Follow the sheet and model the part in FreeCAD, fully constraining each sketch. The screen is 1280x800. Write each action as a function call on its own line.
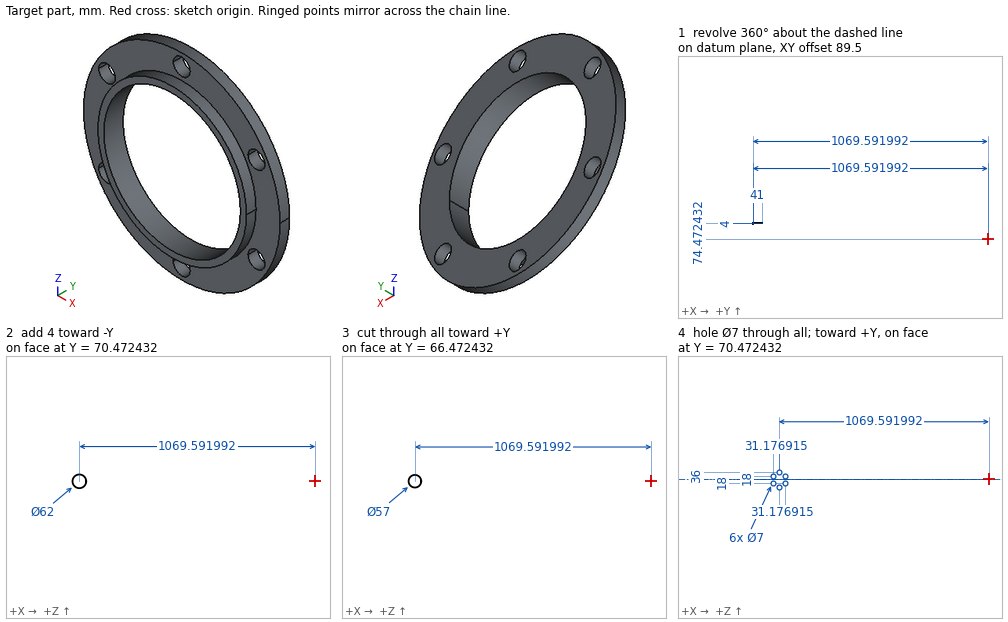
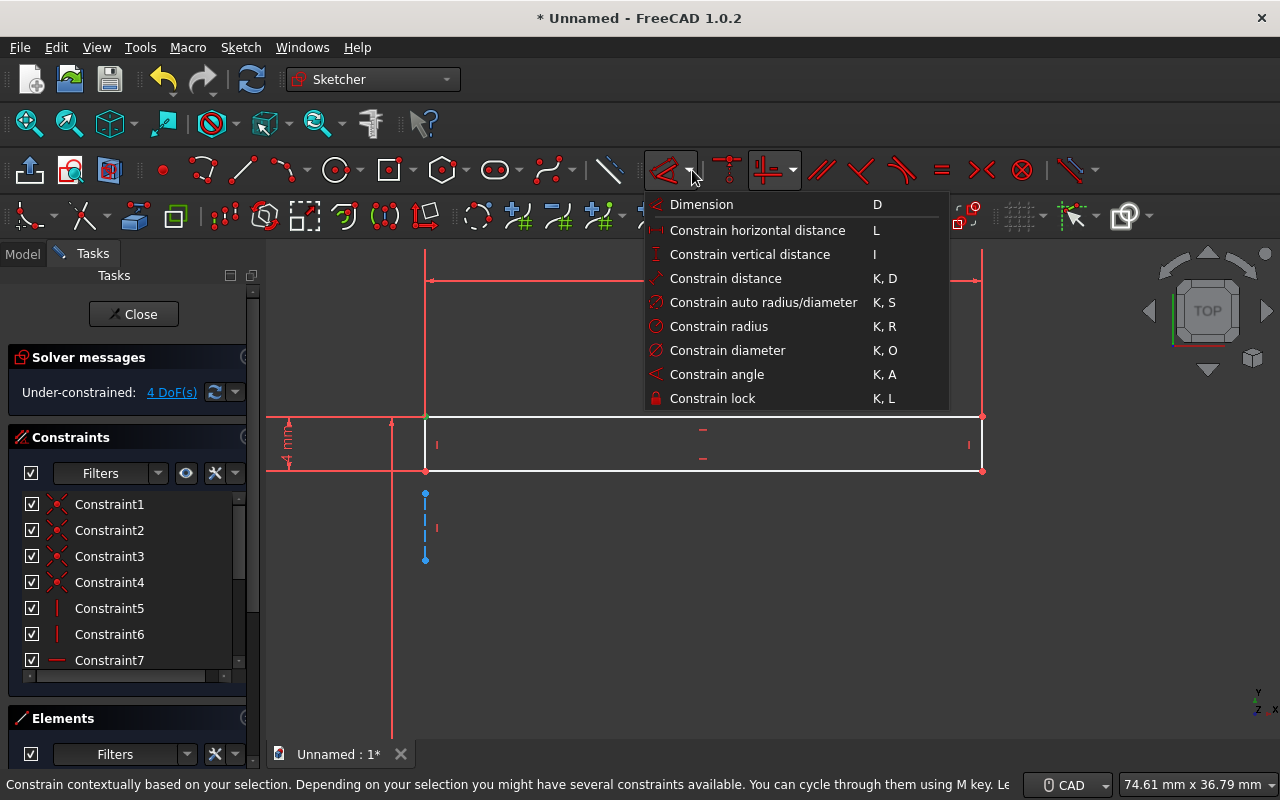
click(797, 230)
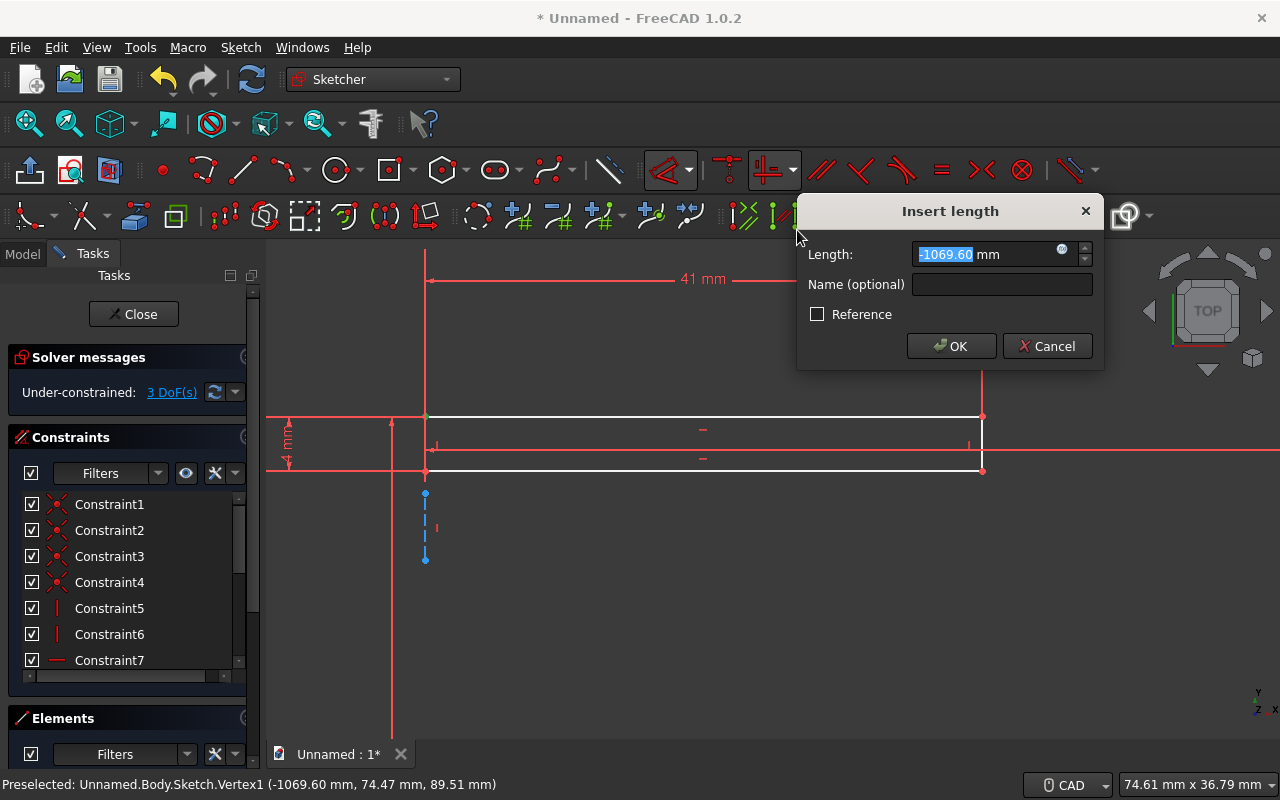
text(-1069.591992)
key(Return)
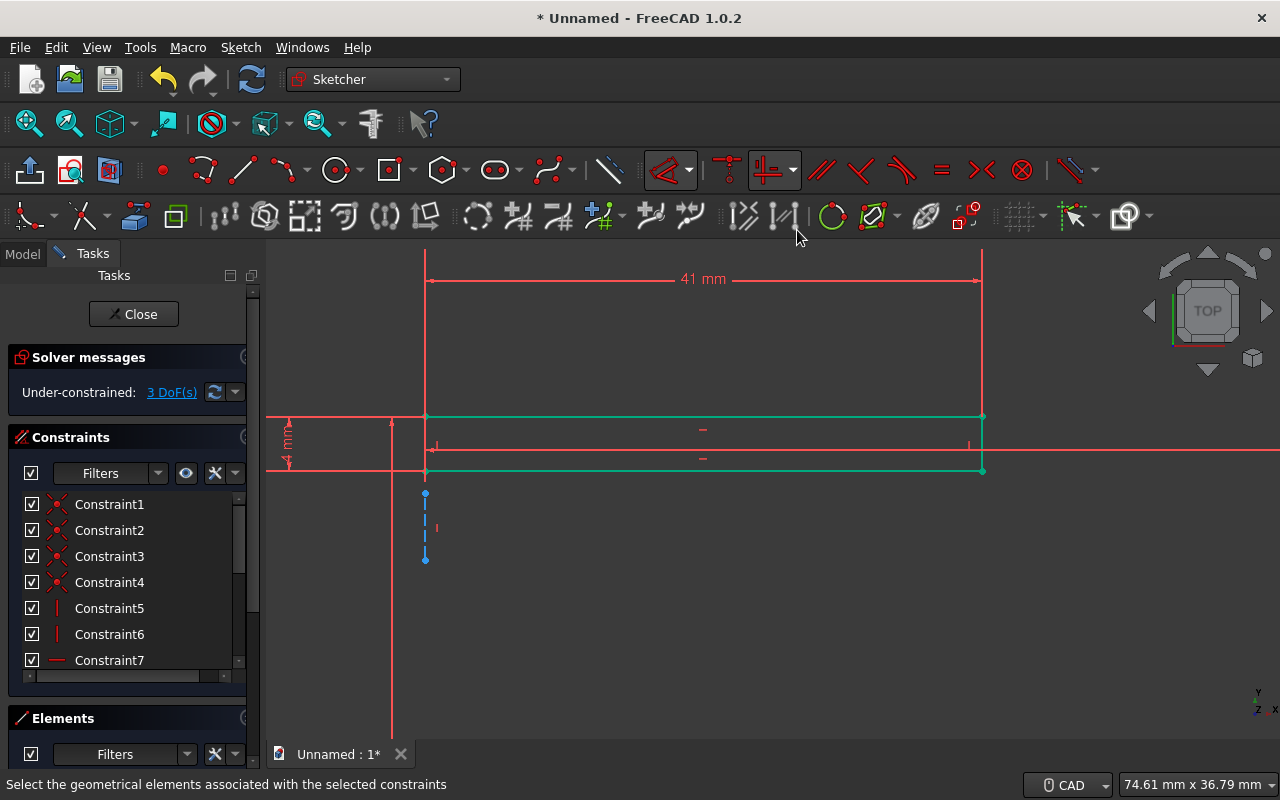
click(425, 494)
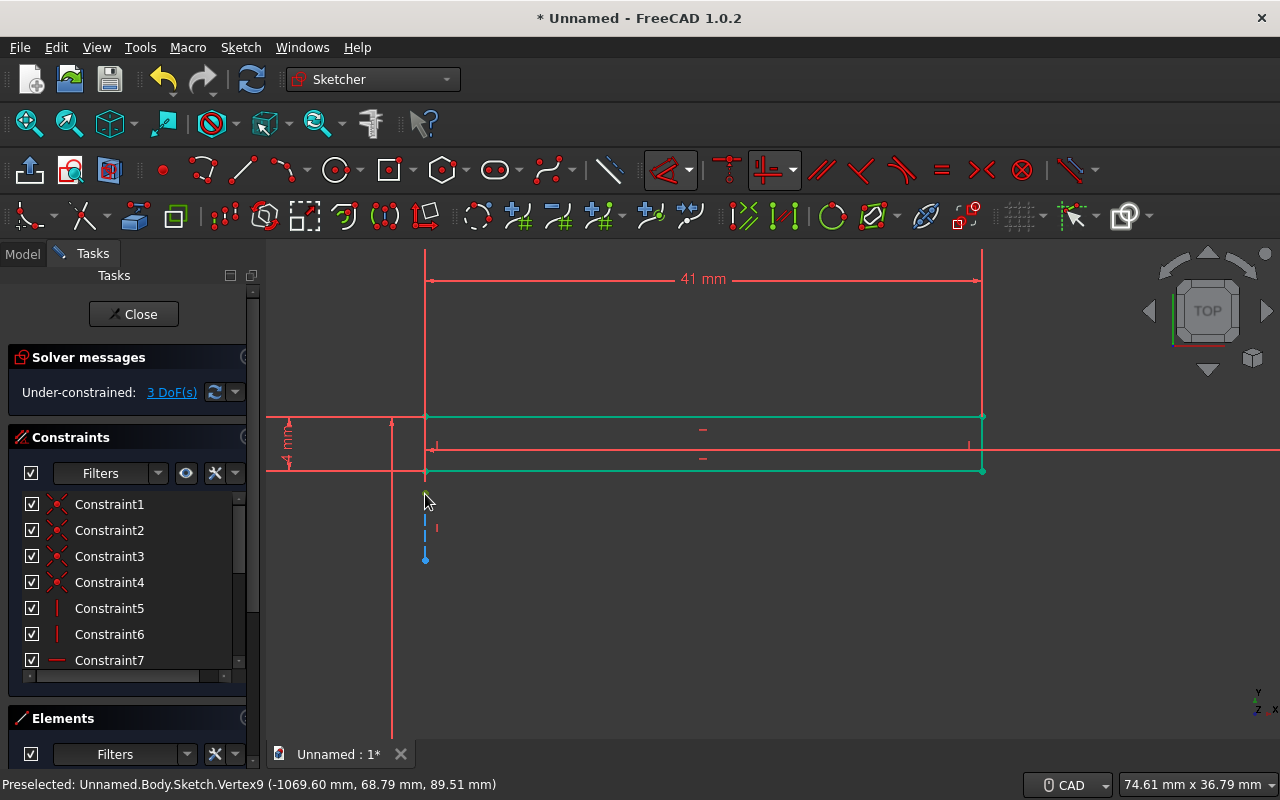
key(l)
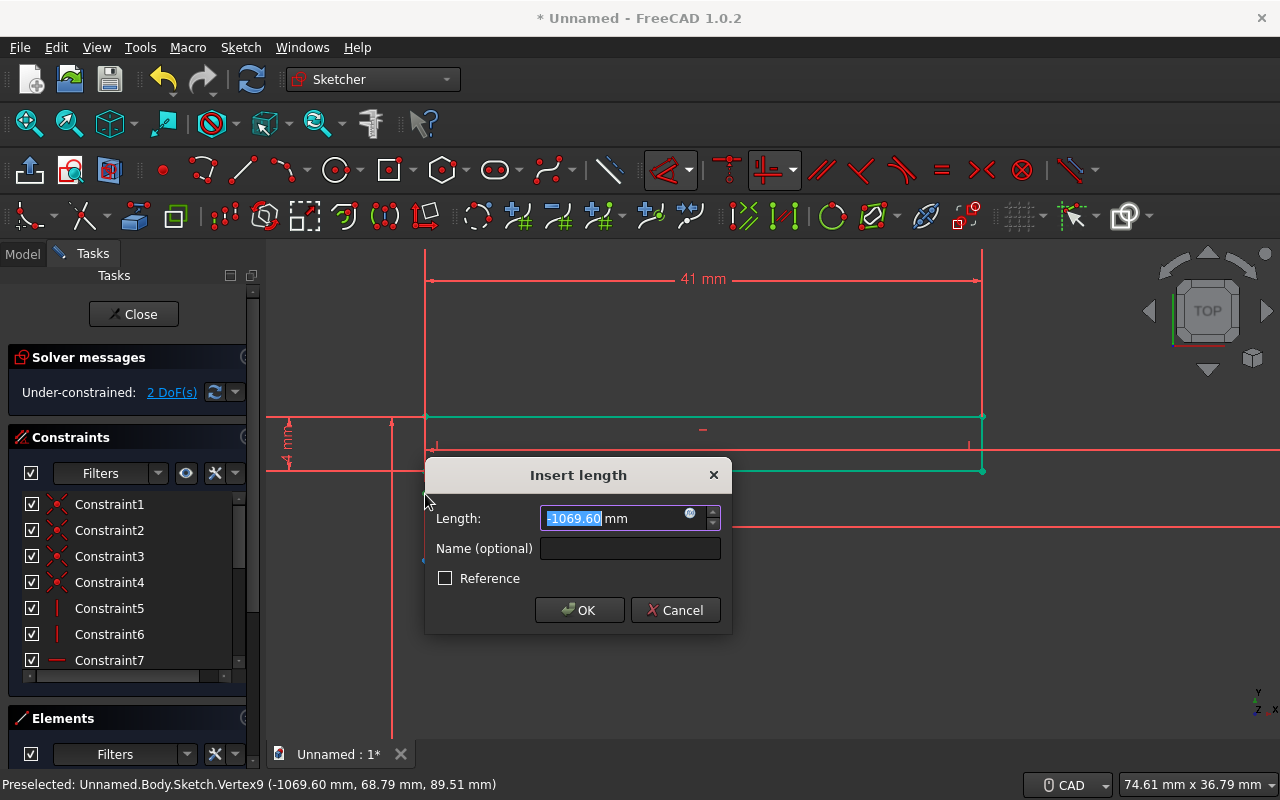
text(-1069.591992)
key(Return)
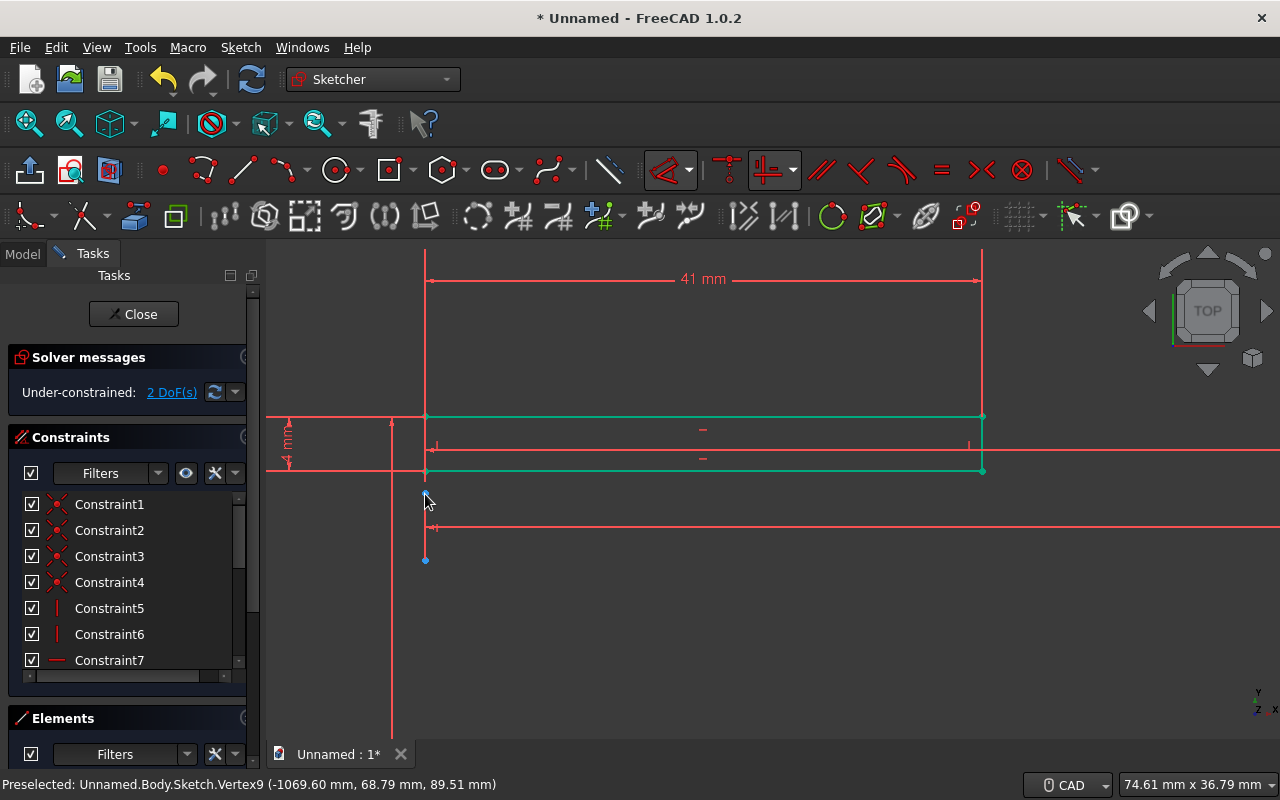
click(134, 314)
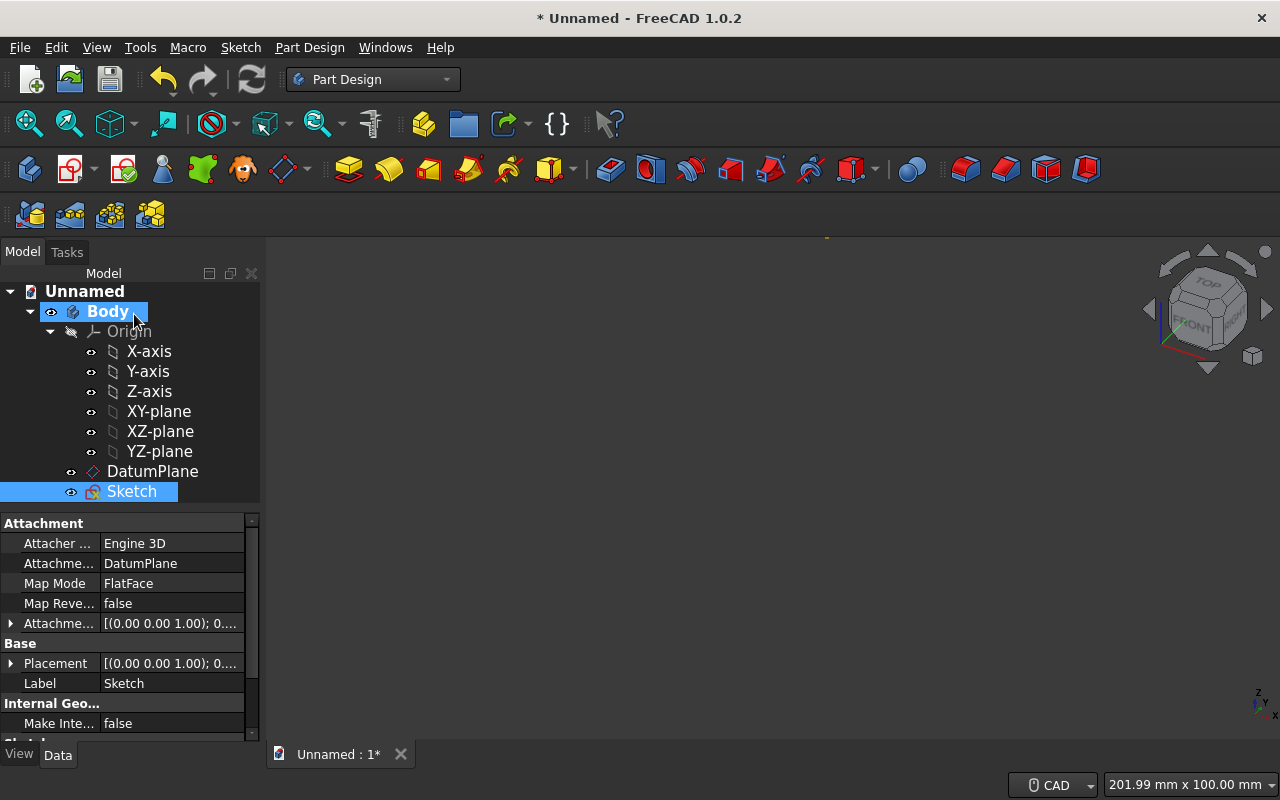
click(390, 170)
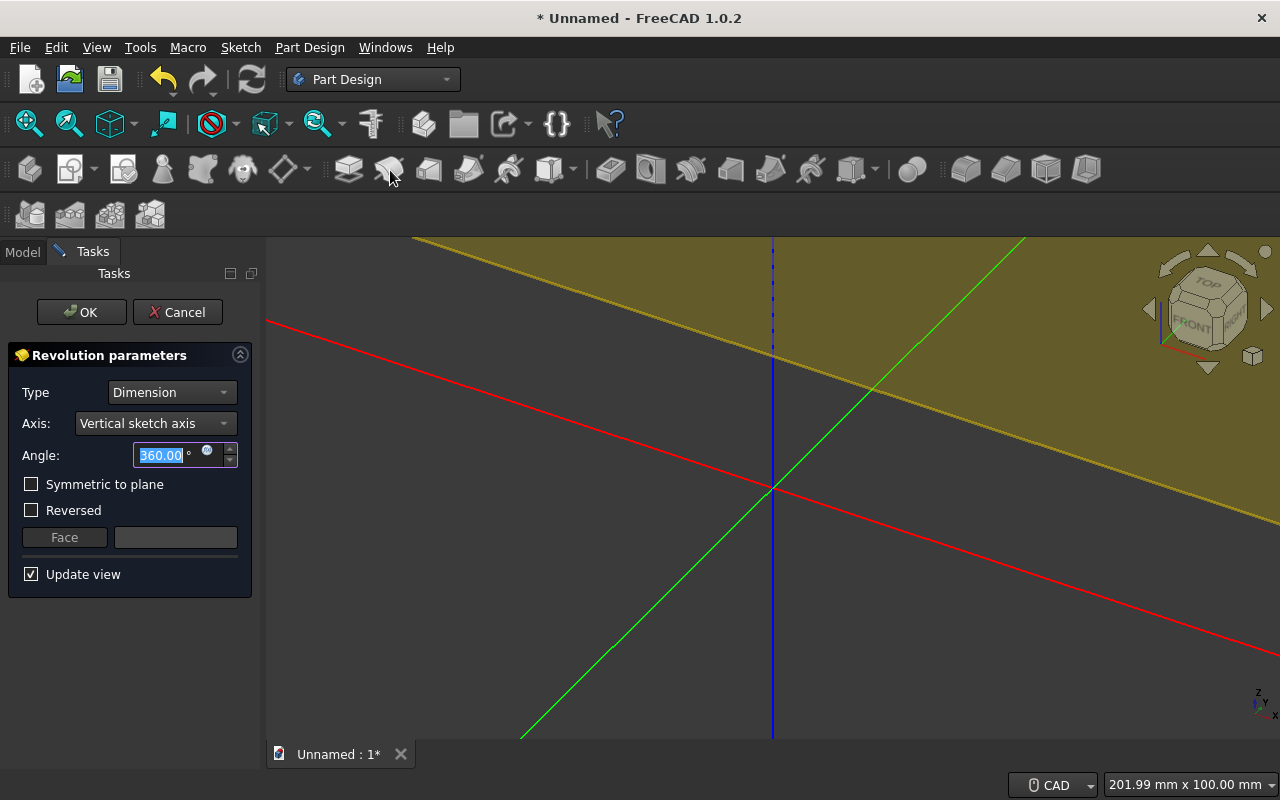
click(156, 424)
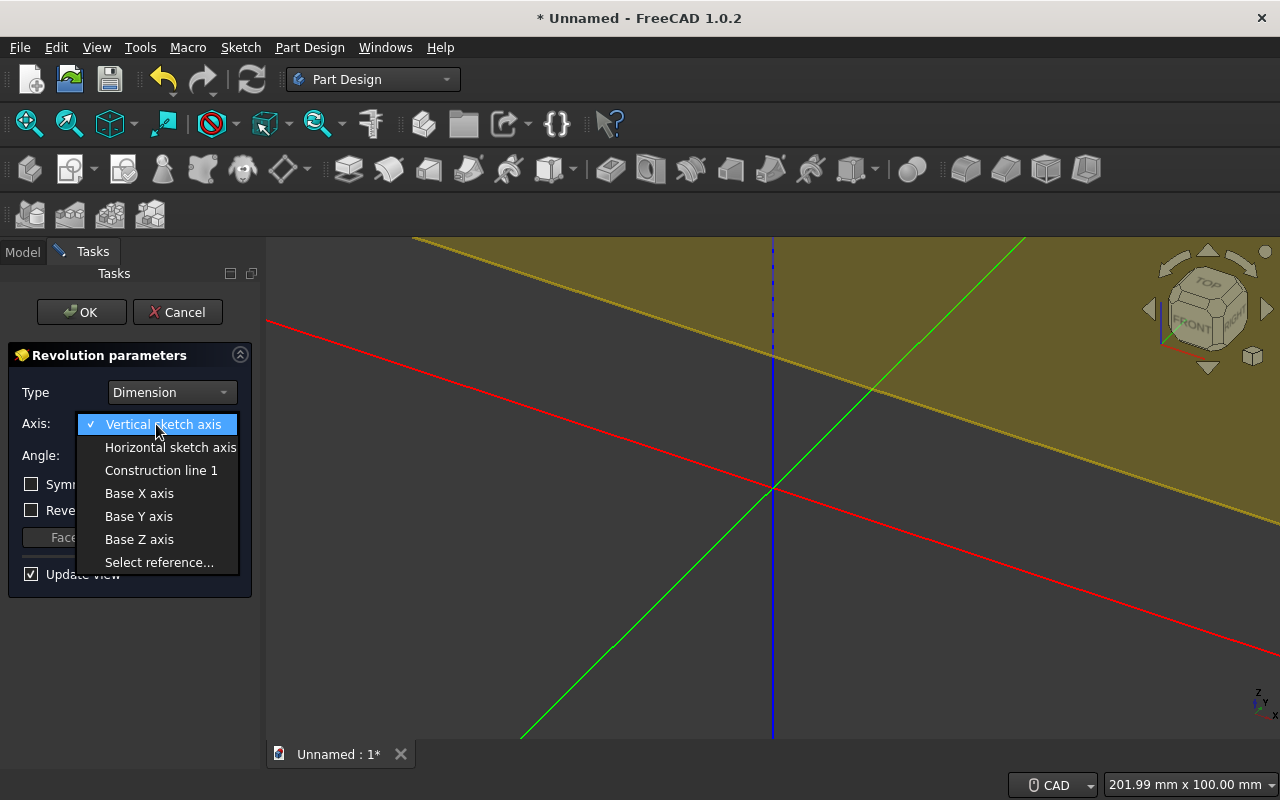
click(156, 470)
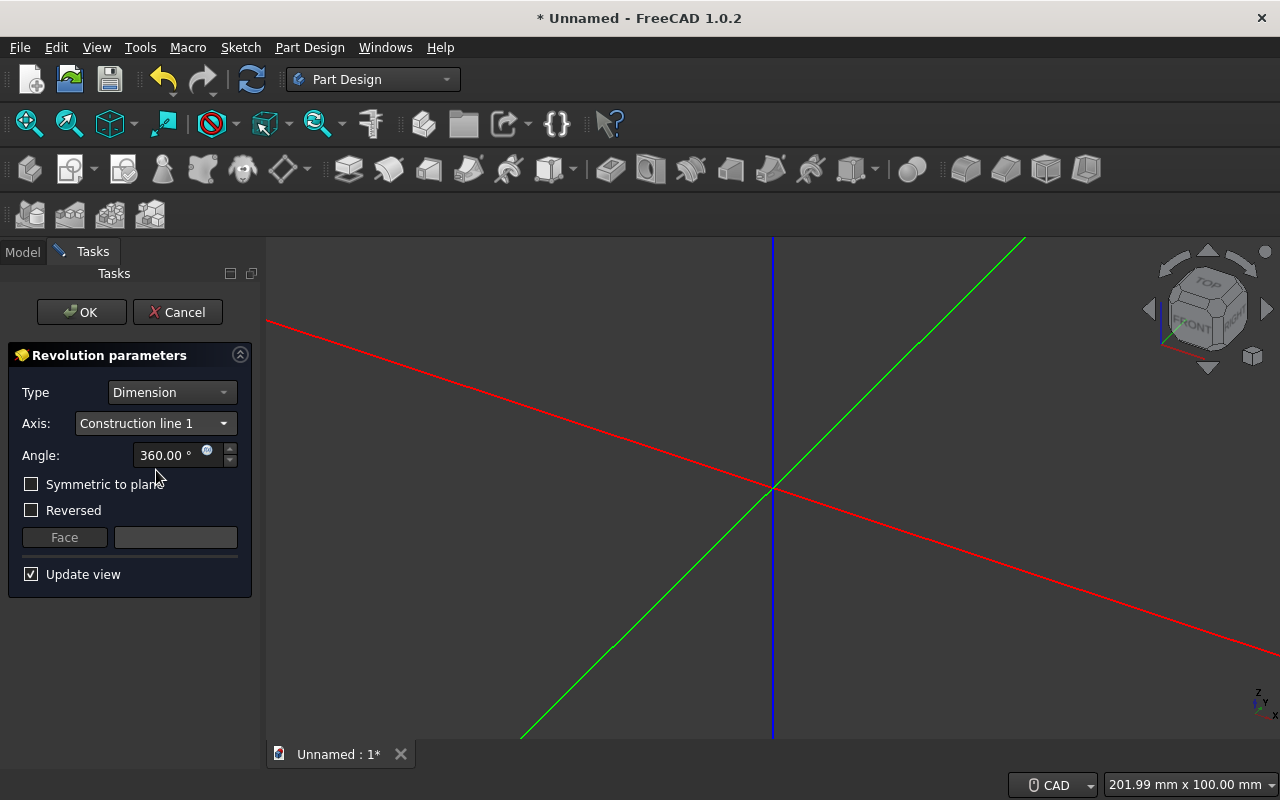
click(82, 312)